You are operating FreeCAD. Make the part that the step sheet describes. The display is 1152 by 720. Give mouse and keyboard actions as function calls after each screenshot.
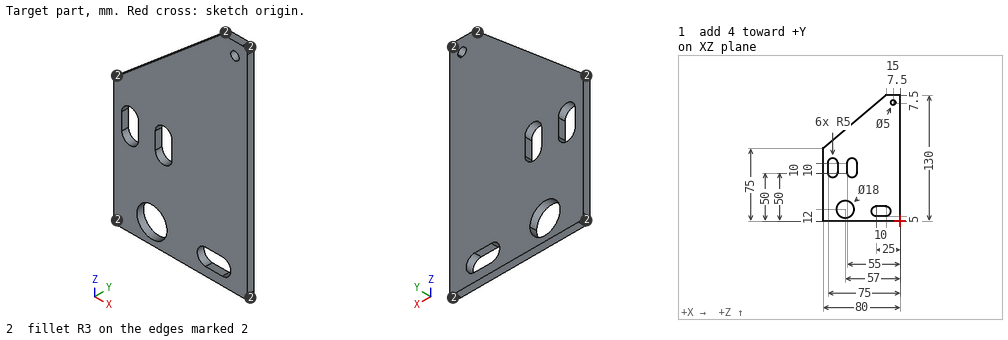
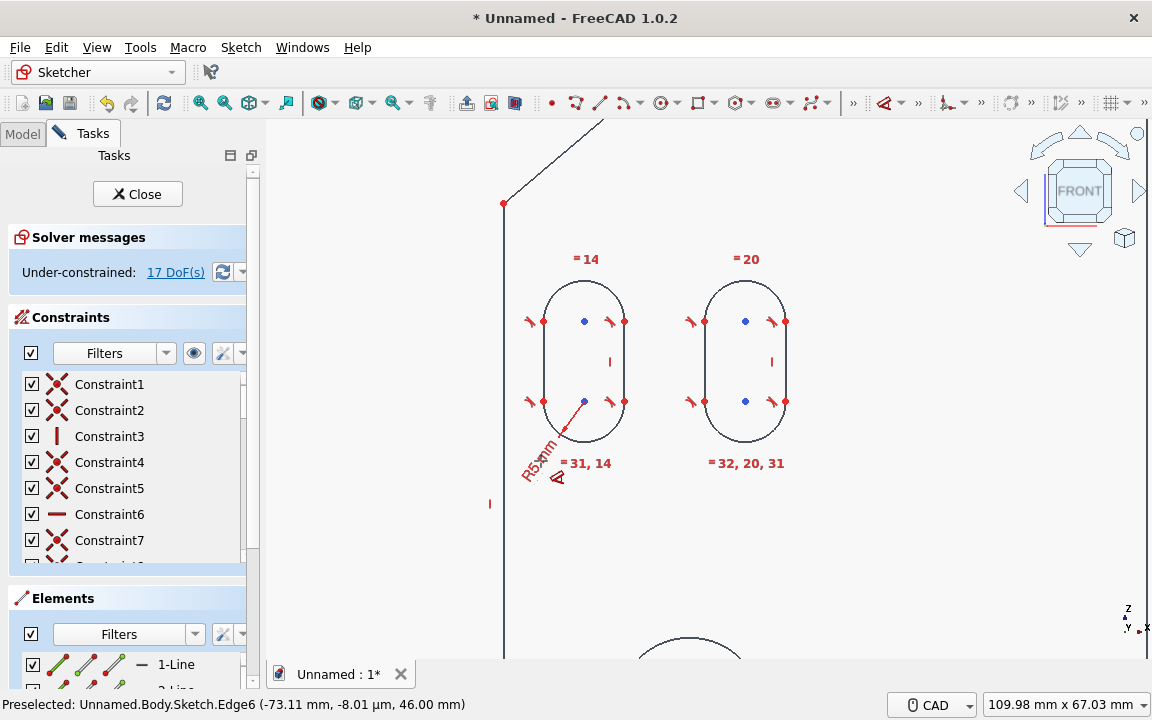
scroll(561, 436, down, 6)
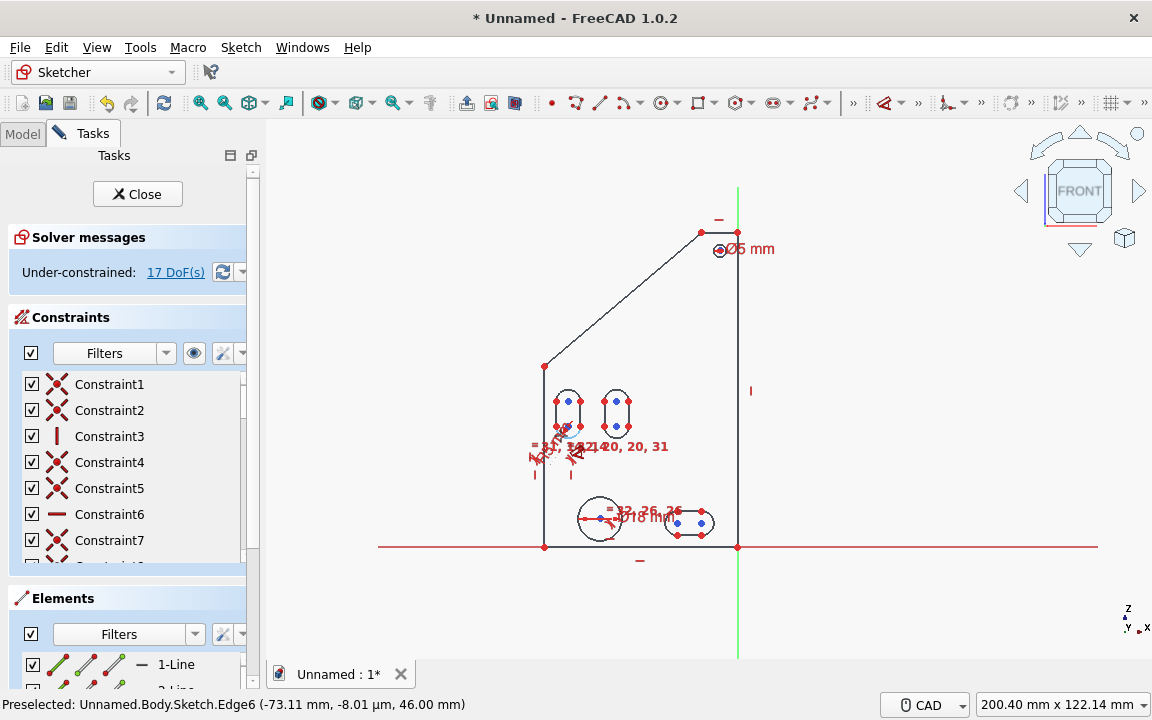
click(680, 547)
click(641, 581)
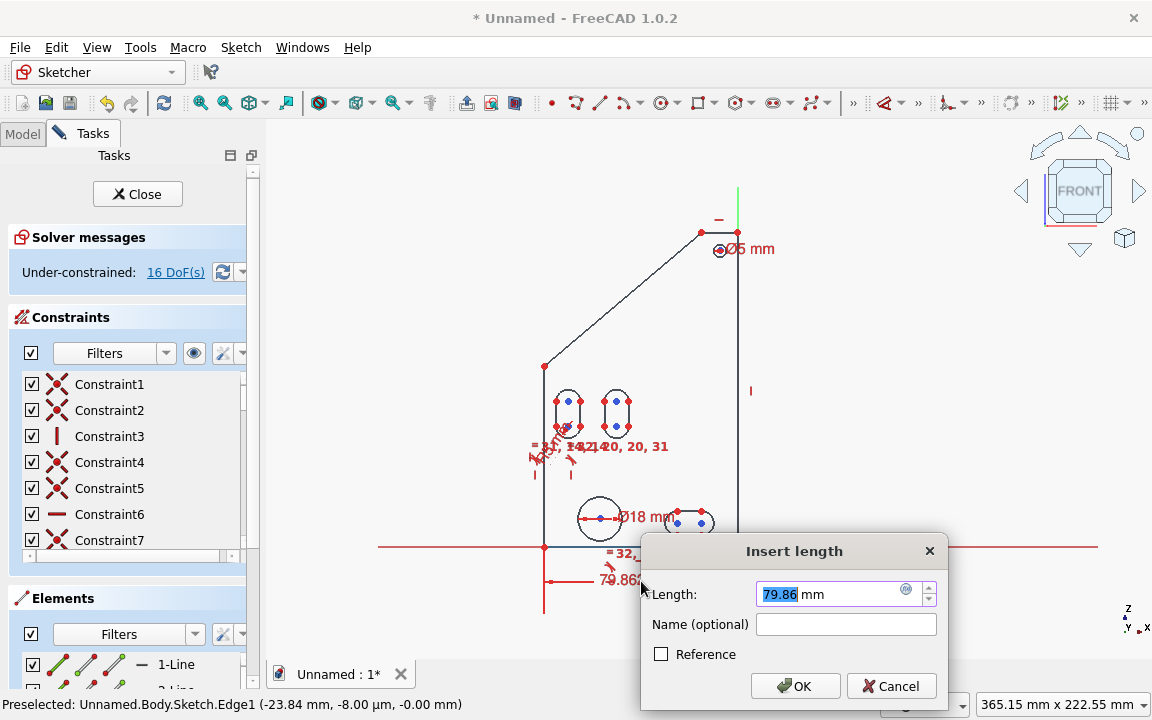
text(80)
key(Return)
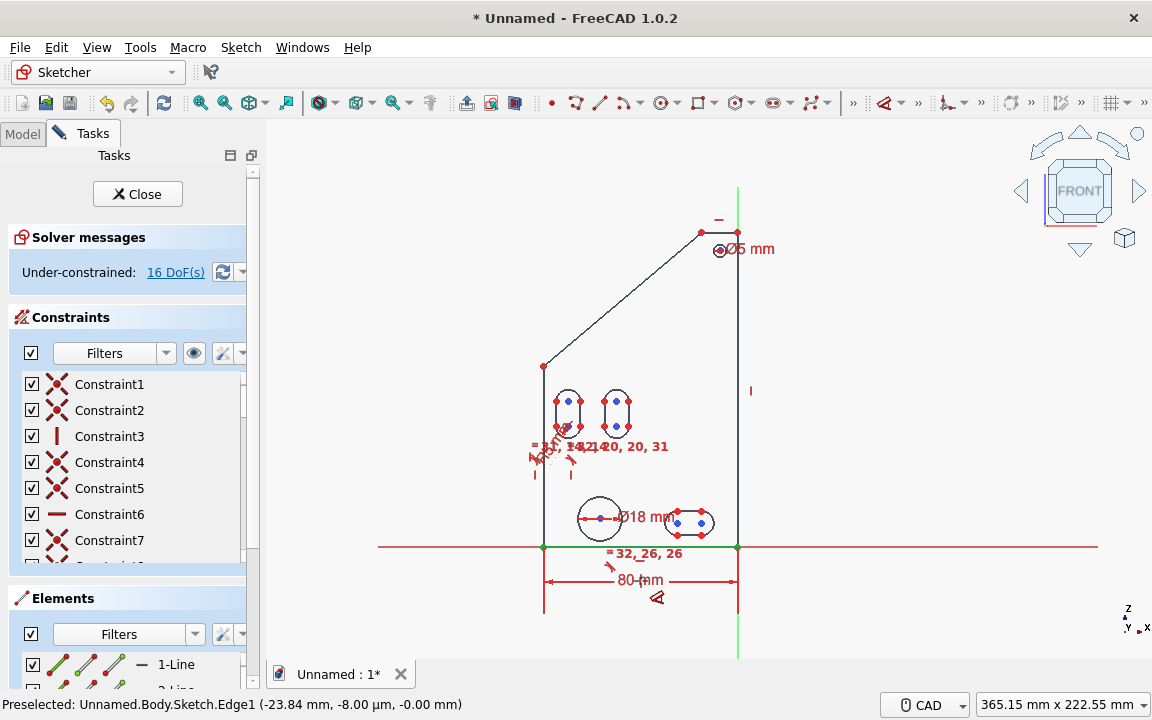
click(544, 493)
click(510, 415)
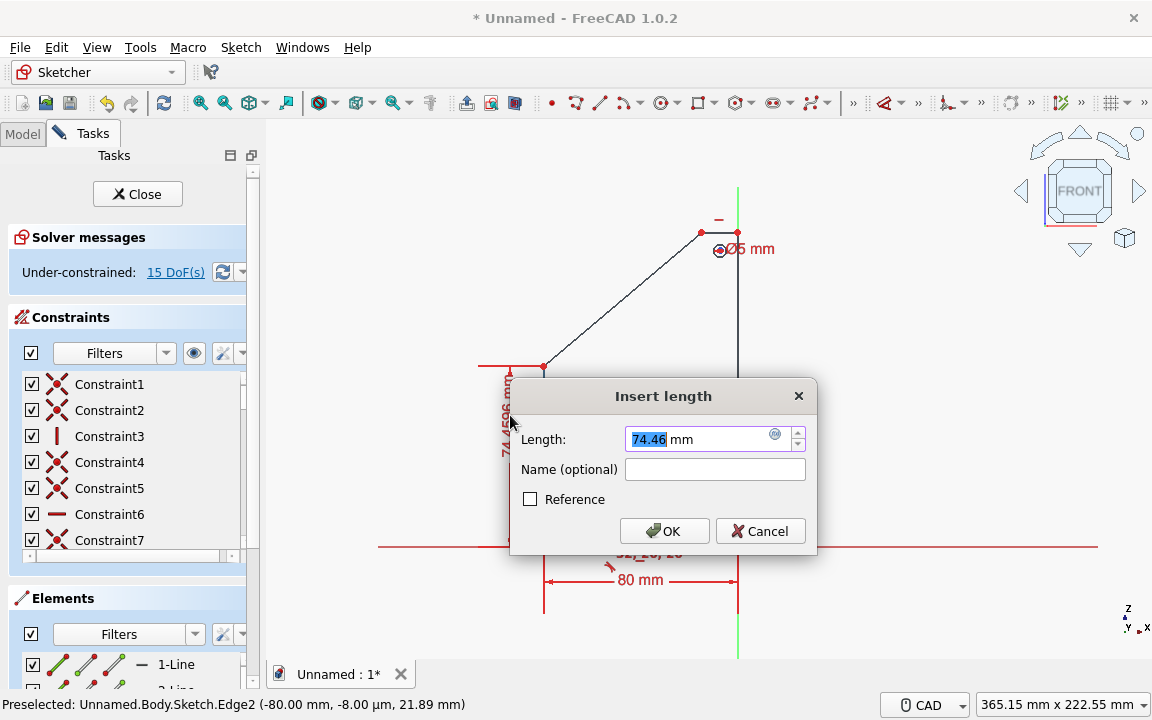
text(75)
key(Return)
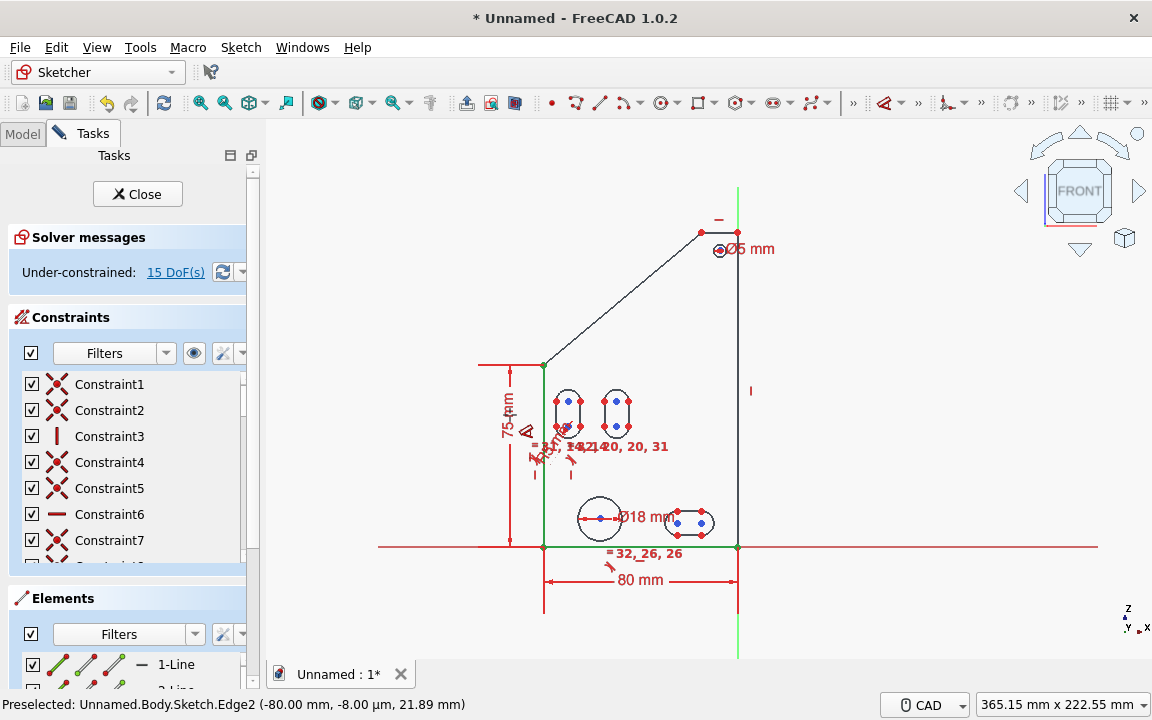
scroll(712, 233, up, 2)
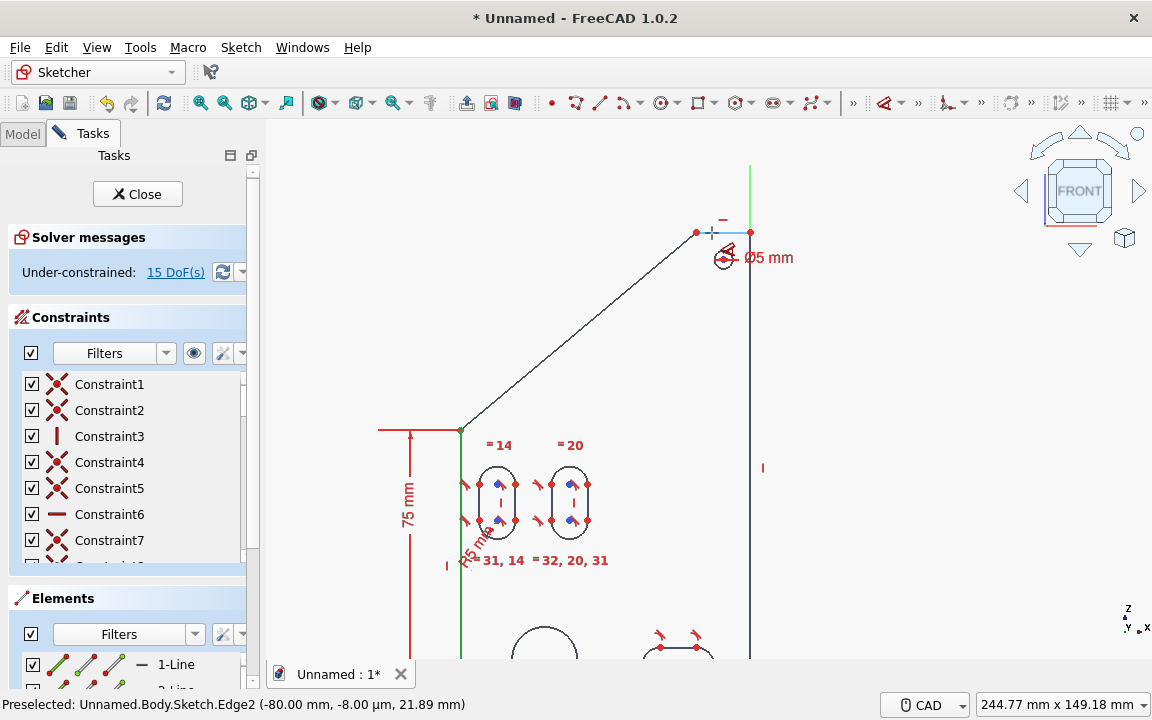
click(712, 233)
click(723, 199)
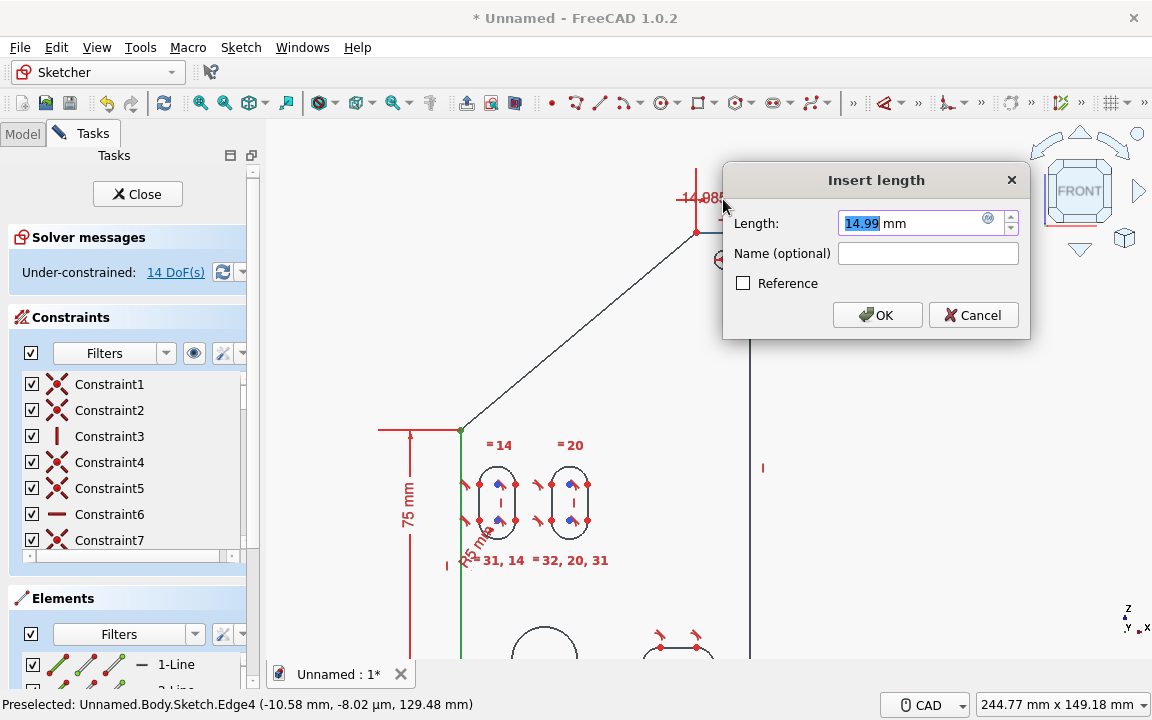
text(15)
key(Return)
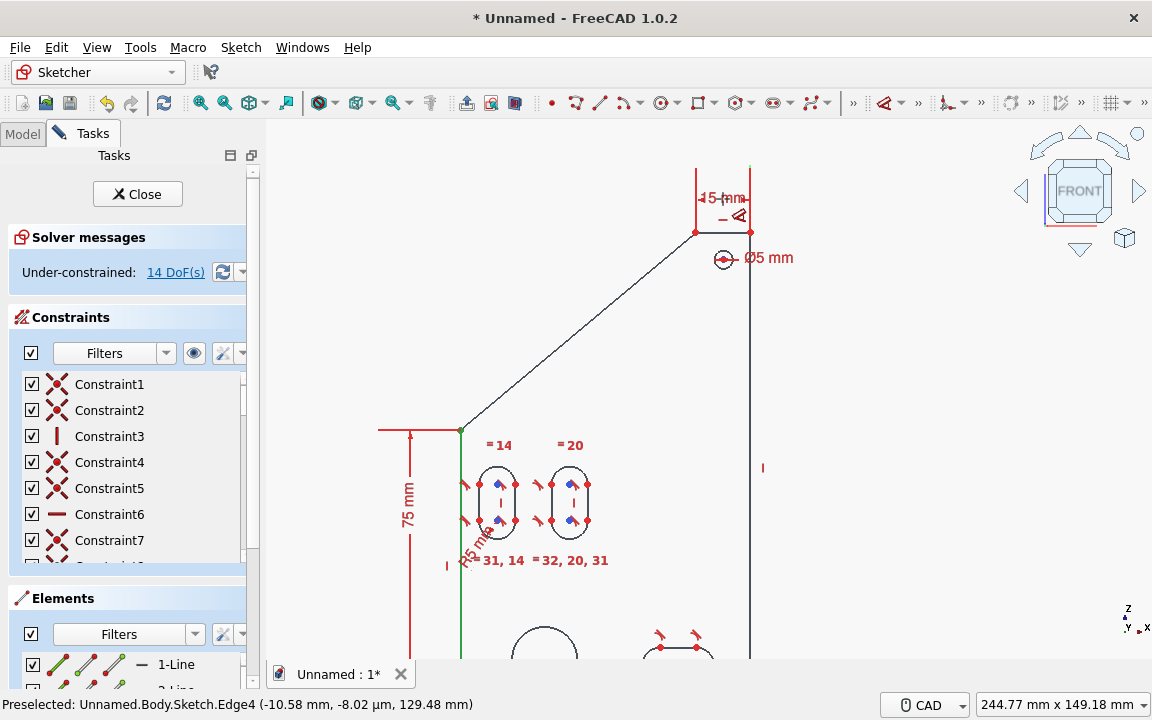
scroll(479, 510, up, 2)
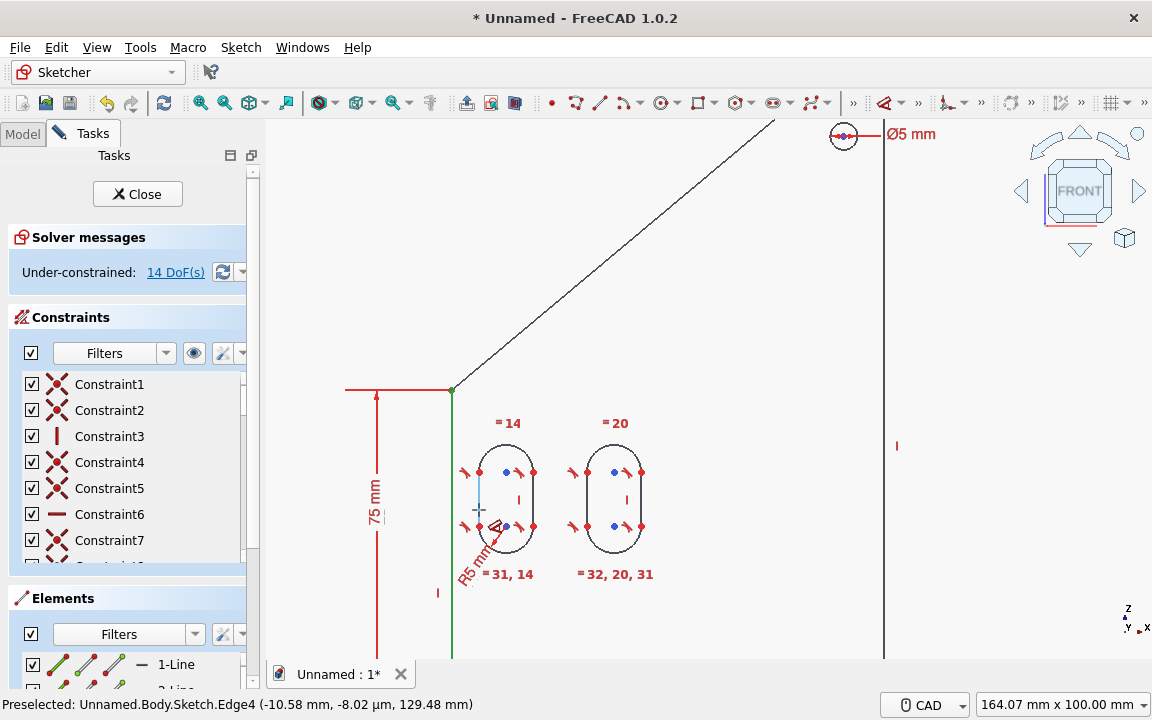
click(479, 510)
click(513, 499)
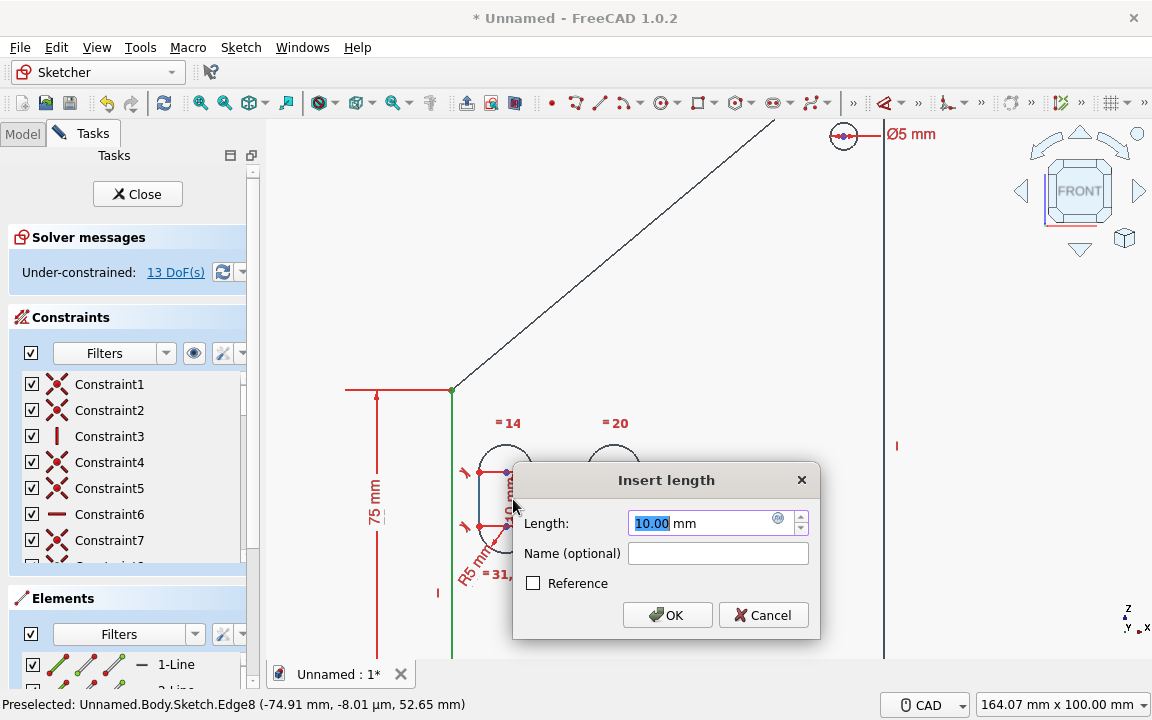
text(10)
key(Return)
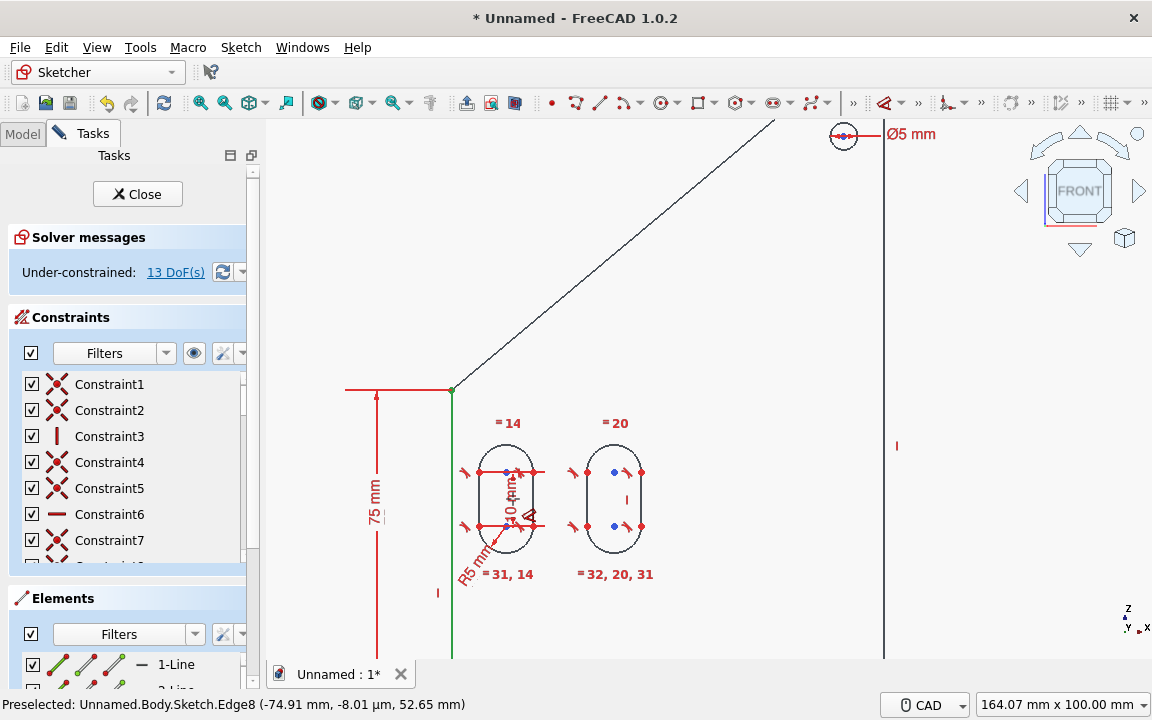
click(587, 510)
click(621, 499)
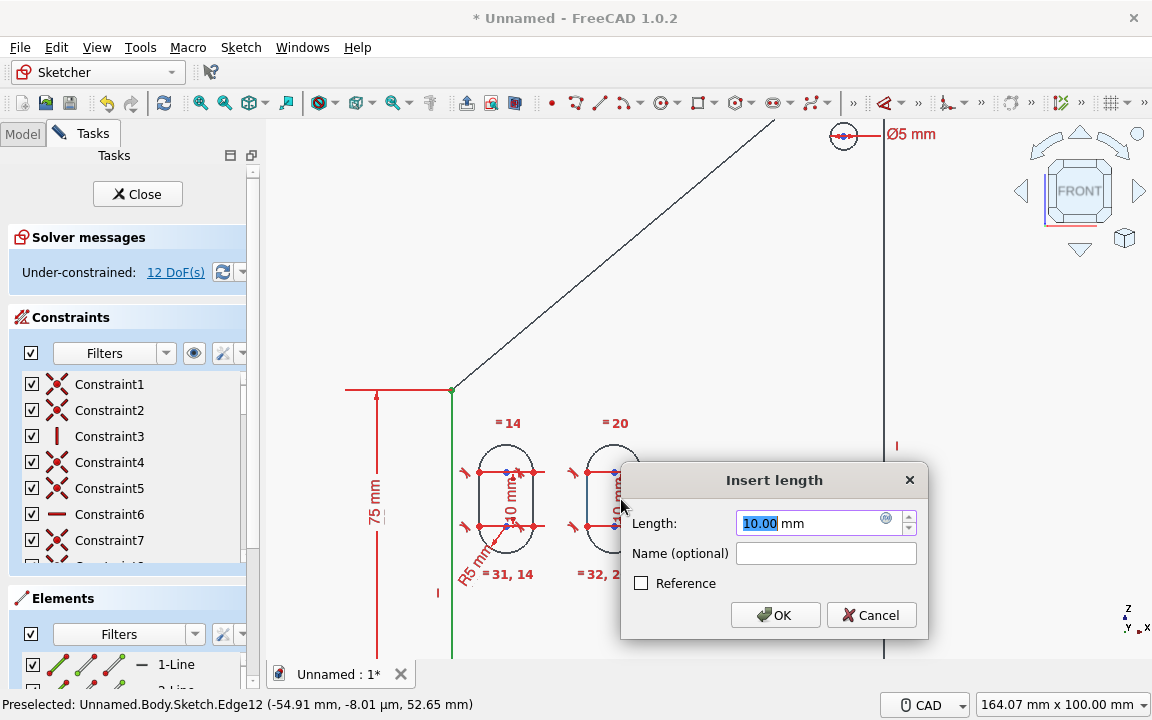
text(10)
key(Return)